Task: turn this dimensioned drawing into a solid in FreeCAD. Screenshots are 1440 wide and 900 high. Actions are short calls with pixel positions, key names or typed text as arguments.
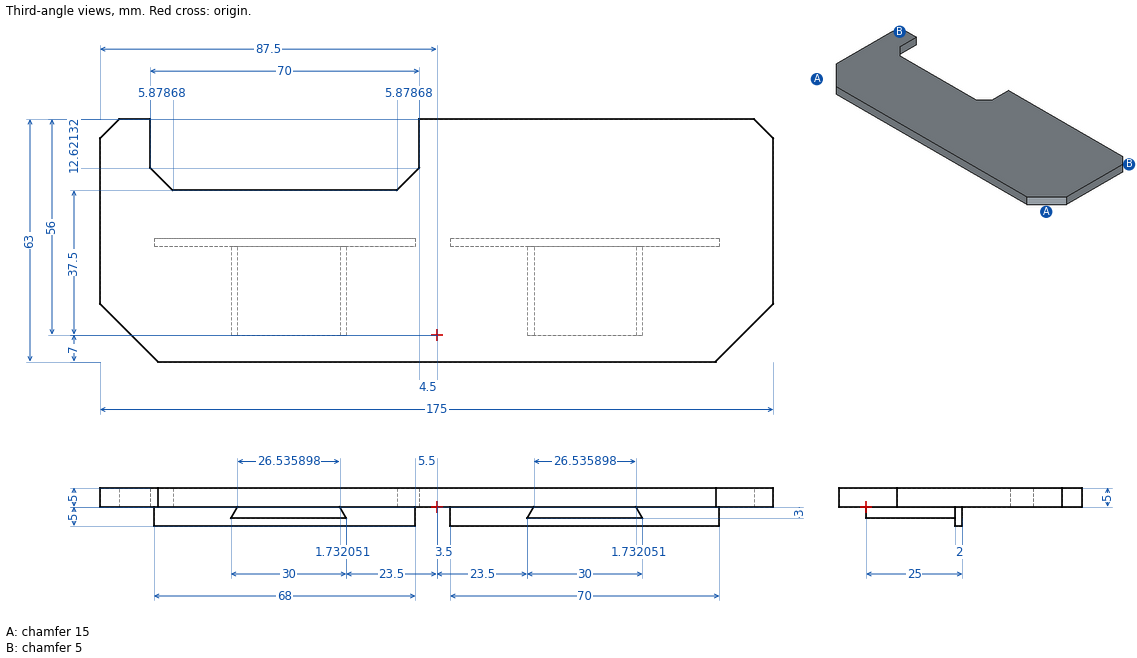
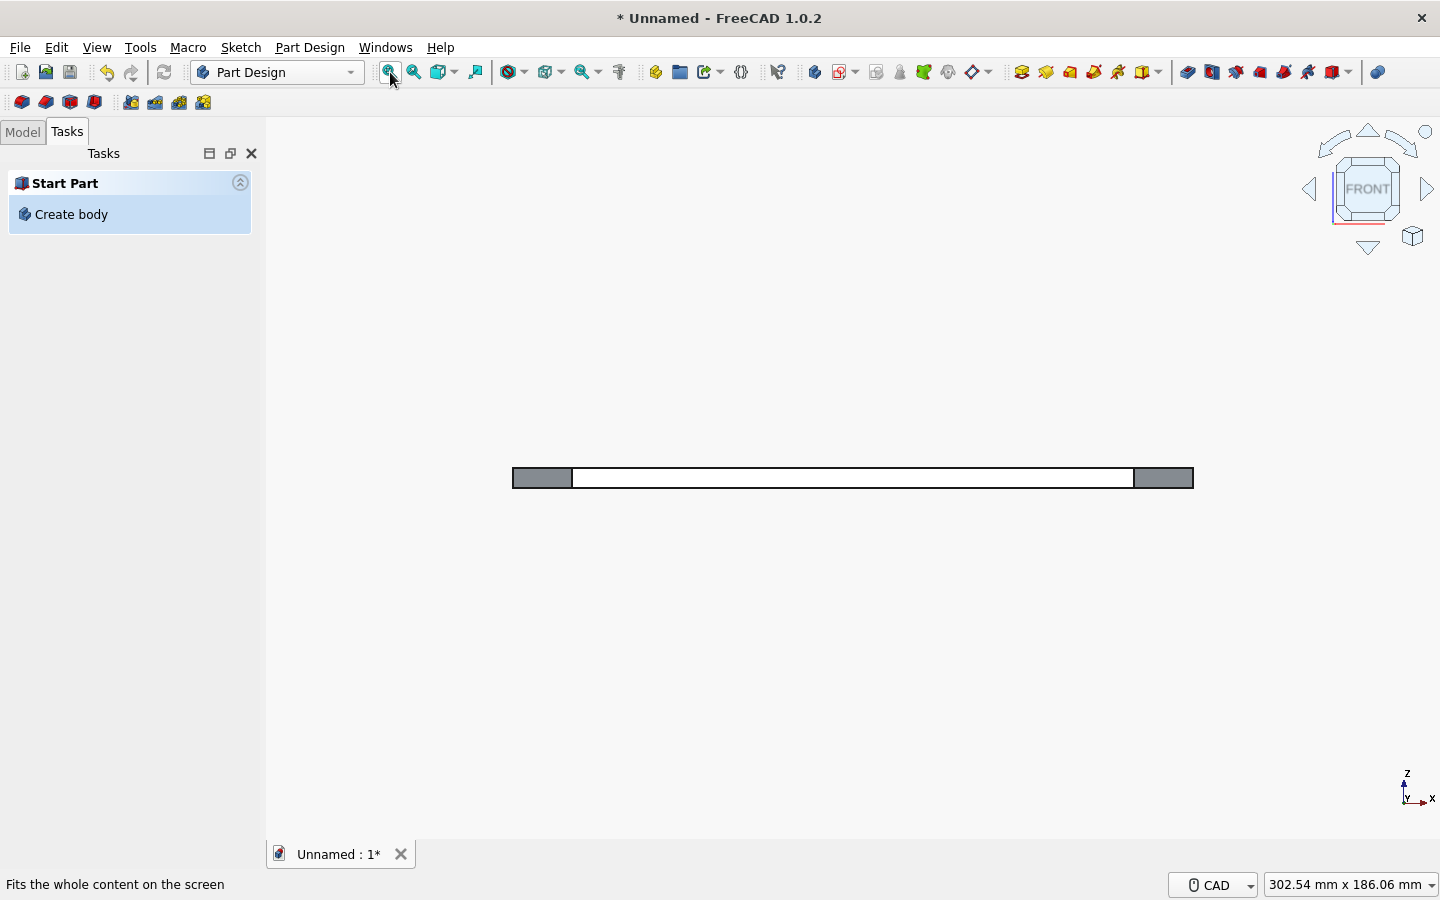
scroll(513, 477, up, 4)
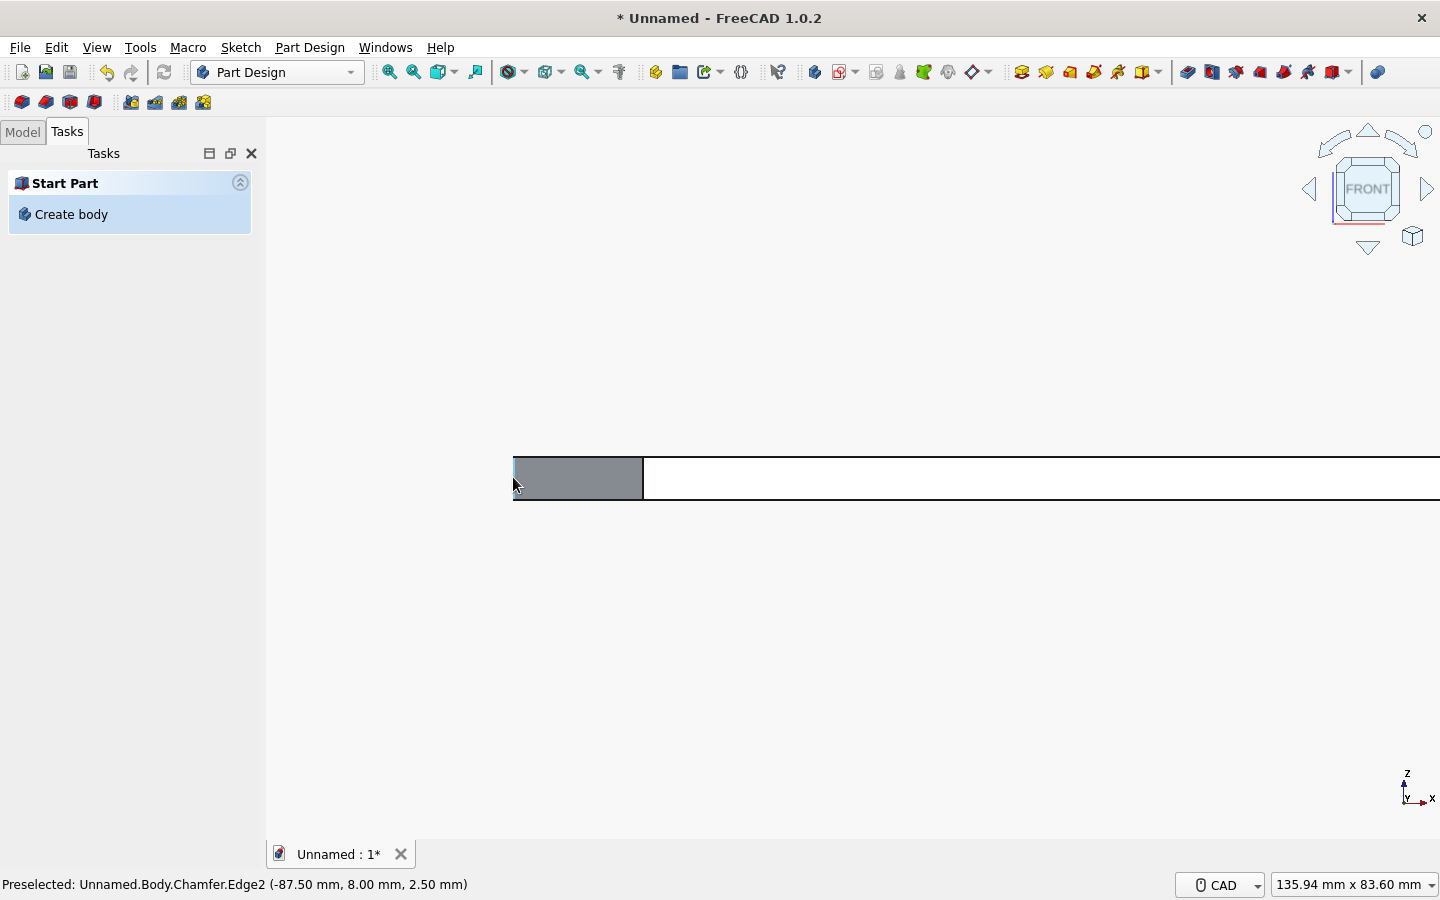
key(v)
key(f)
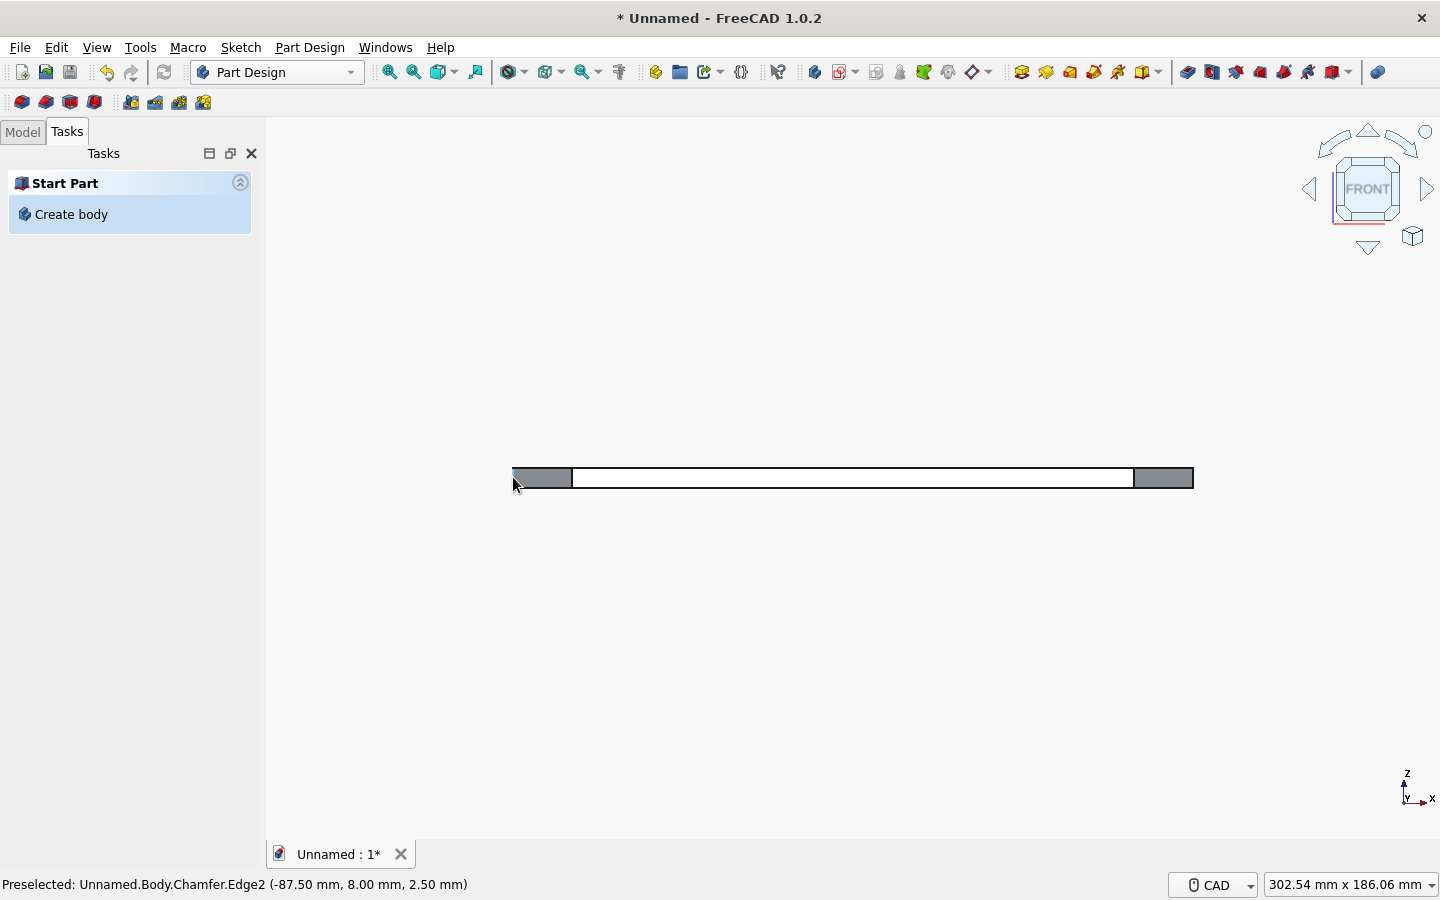
key(3)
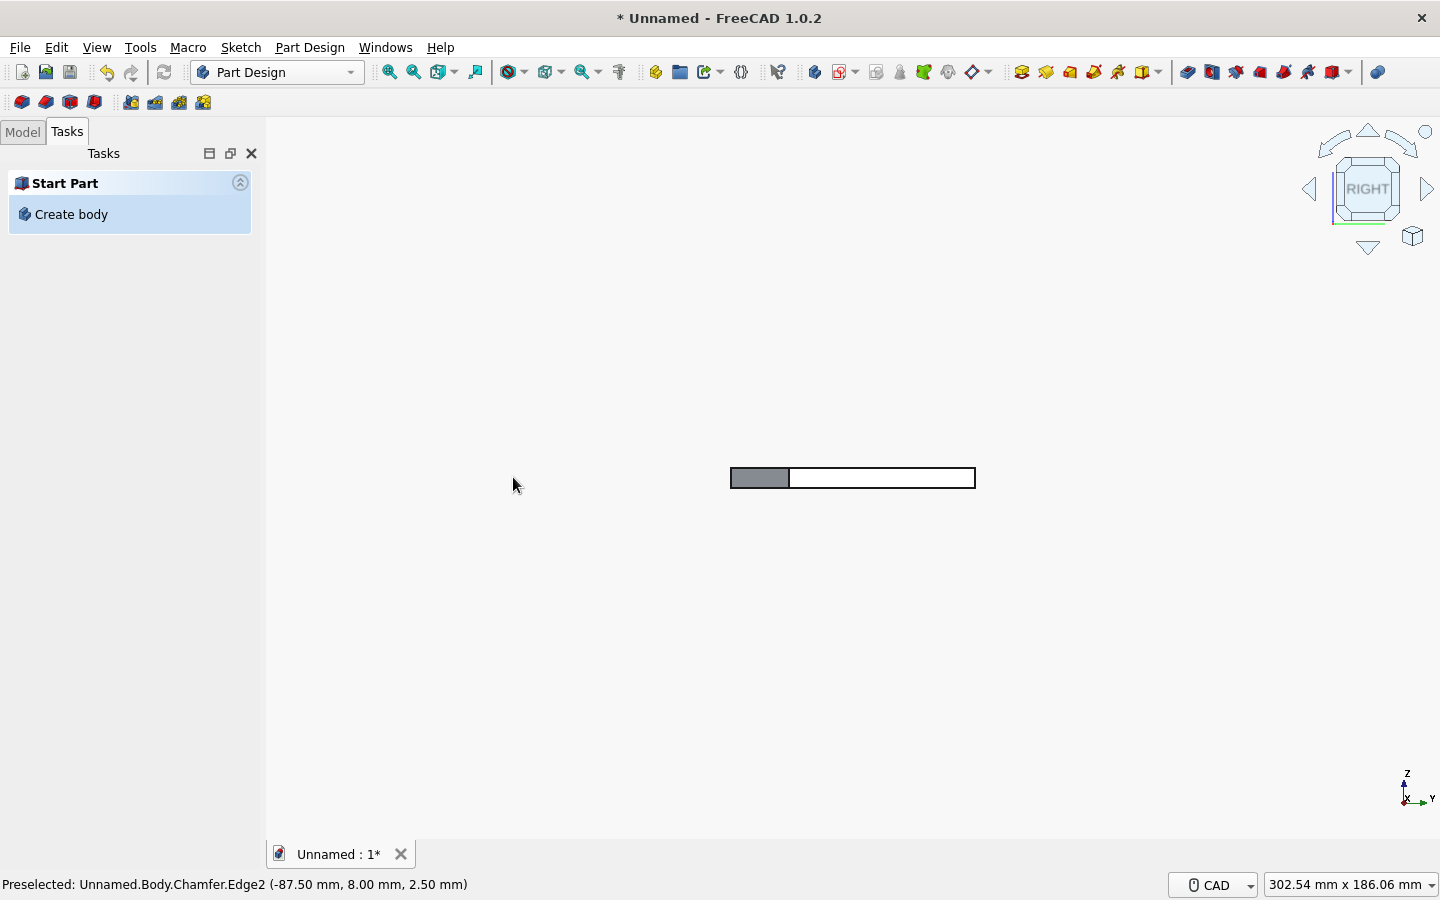
click(390, 72)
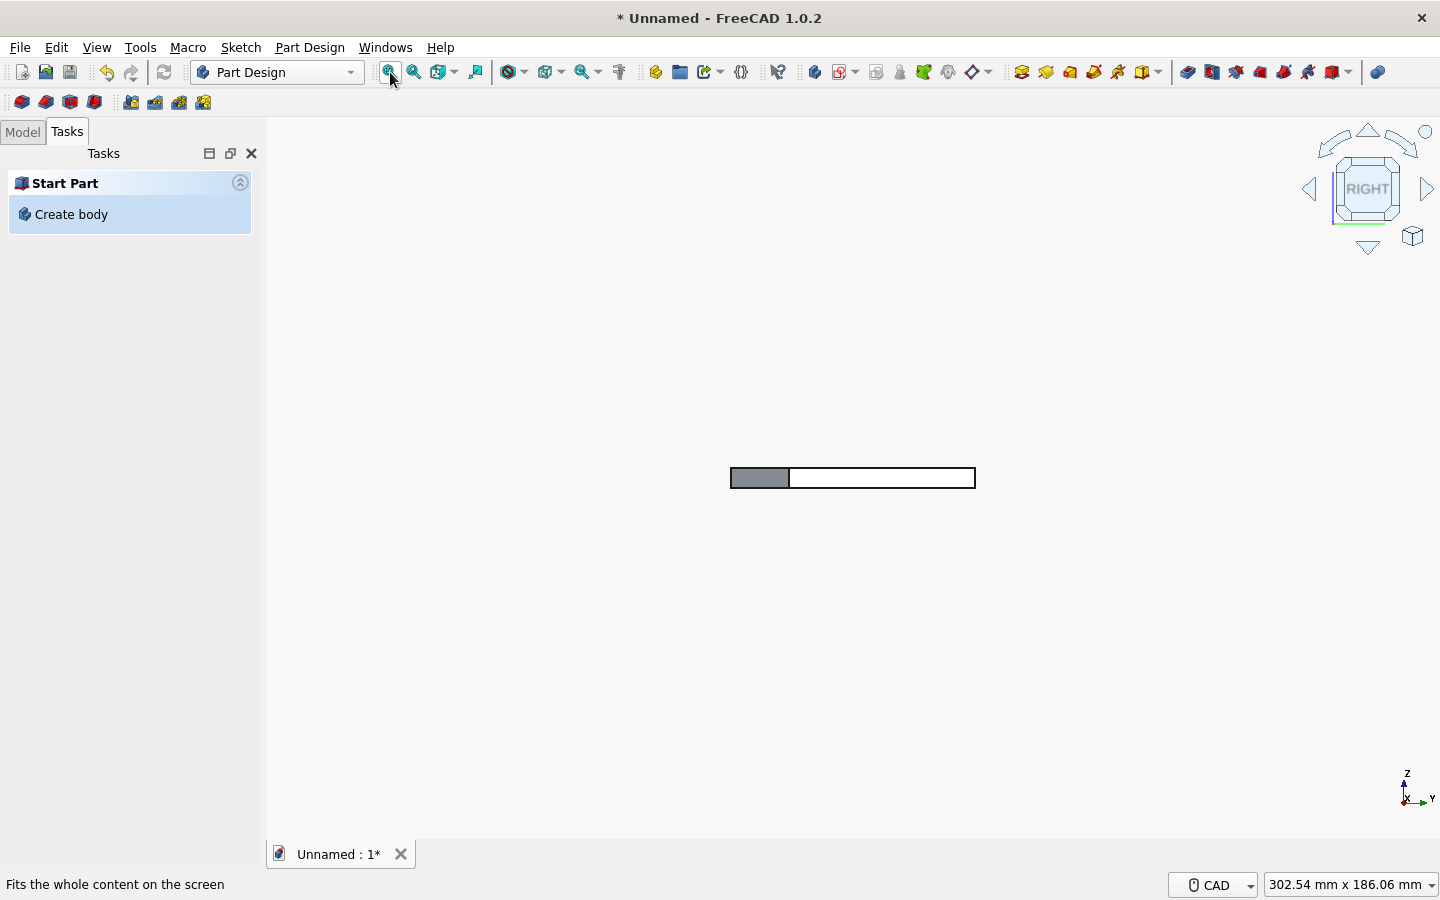
click(975, 477)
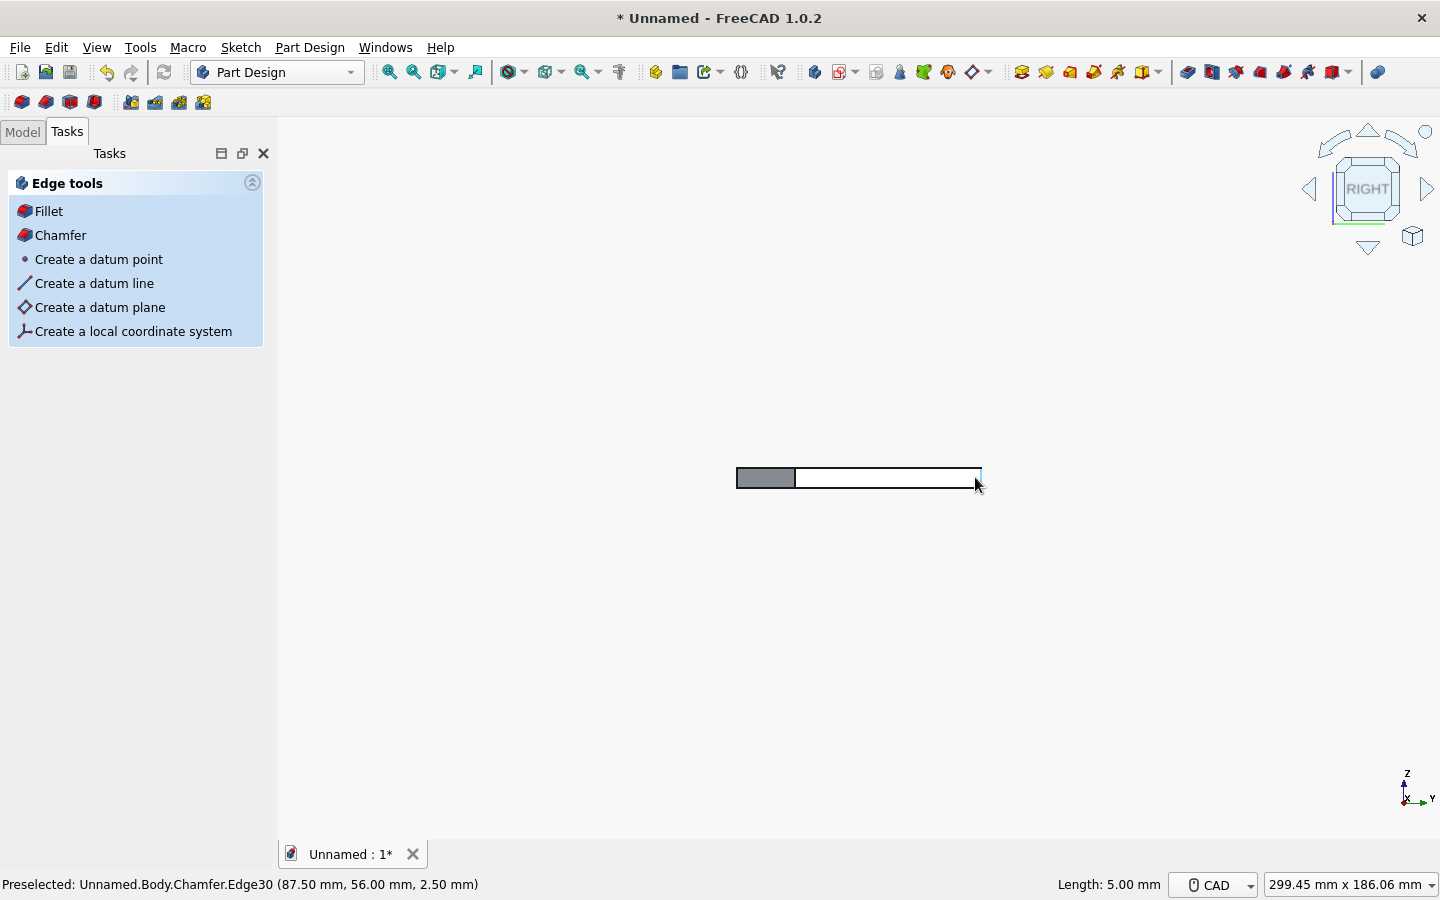
scroll(981, 477, up, 4)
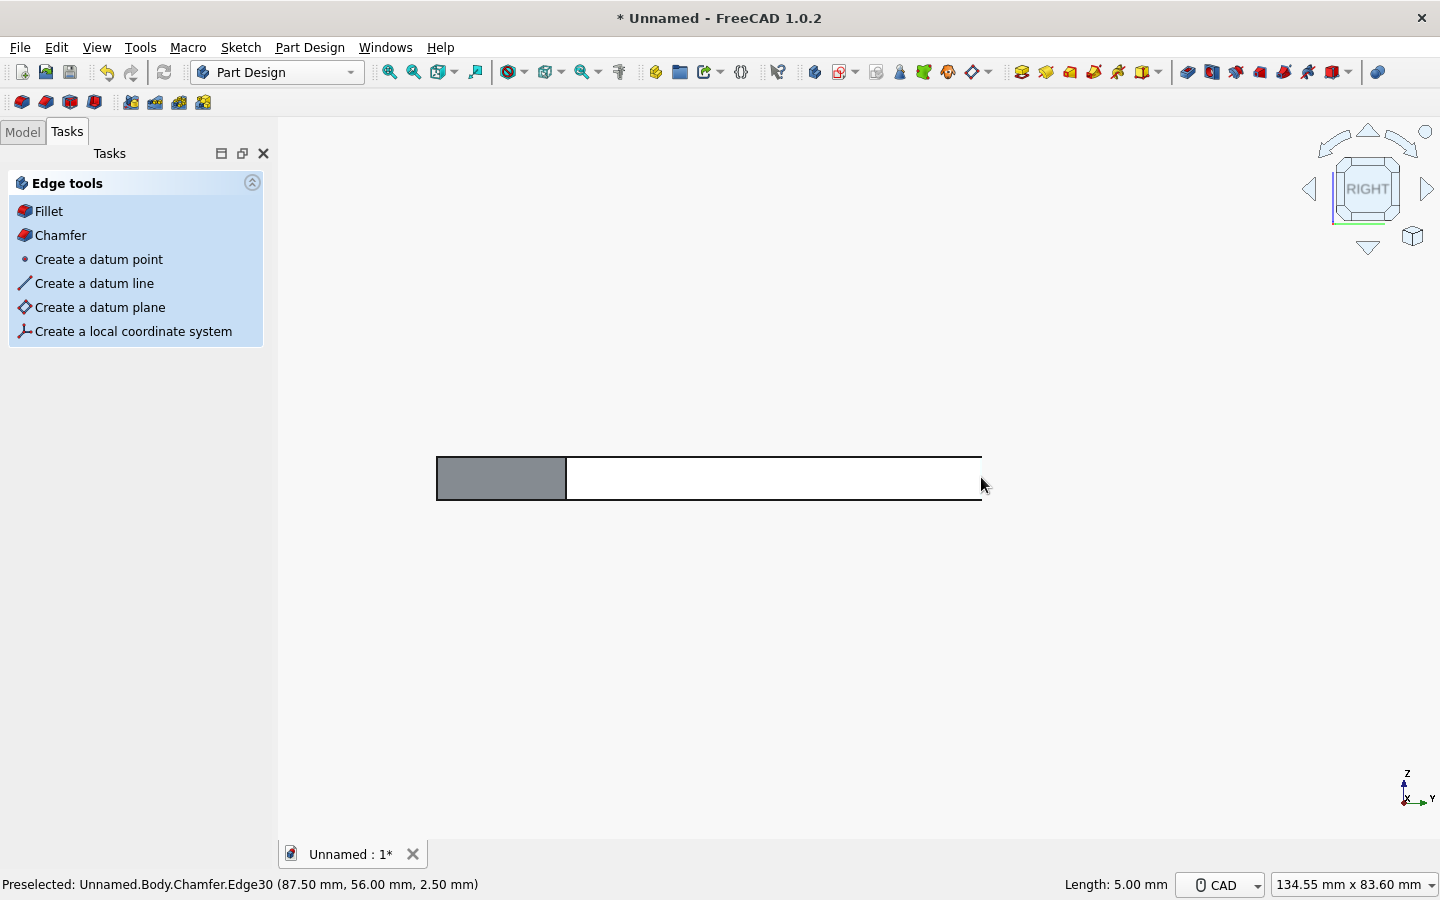
click(390, 72)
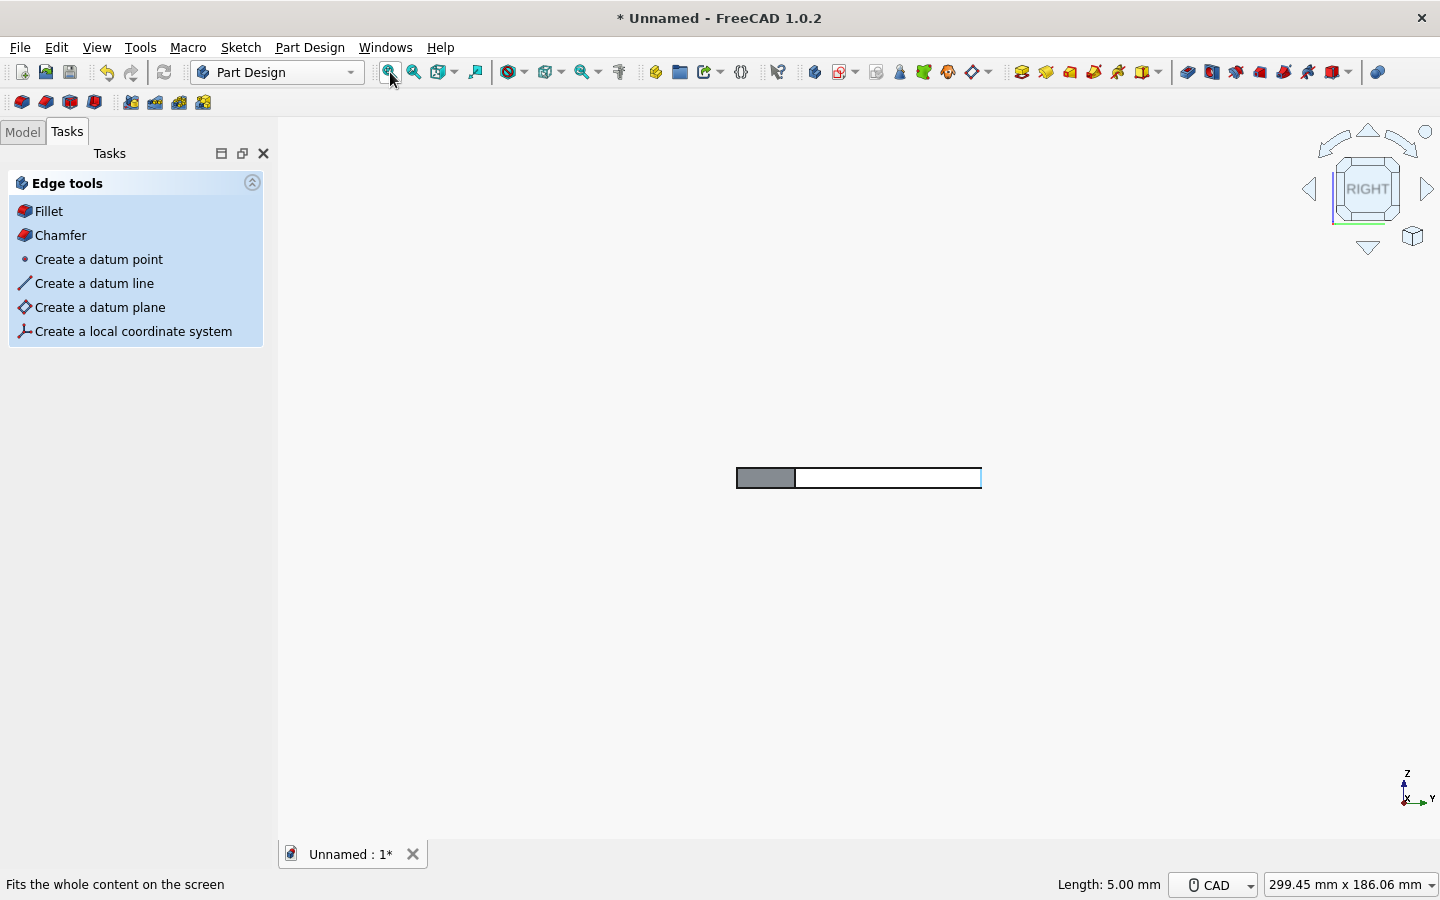
key(5)